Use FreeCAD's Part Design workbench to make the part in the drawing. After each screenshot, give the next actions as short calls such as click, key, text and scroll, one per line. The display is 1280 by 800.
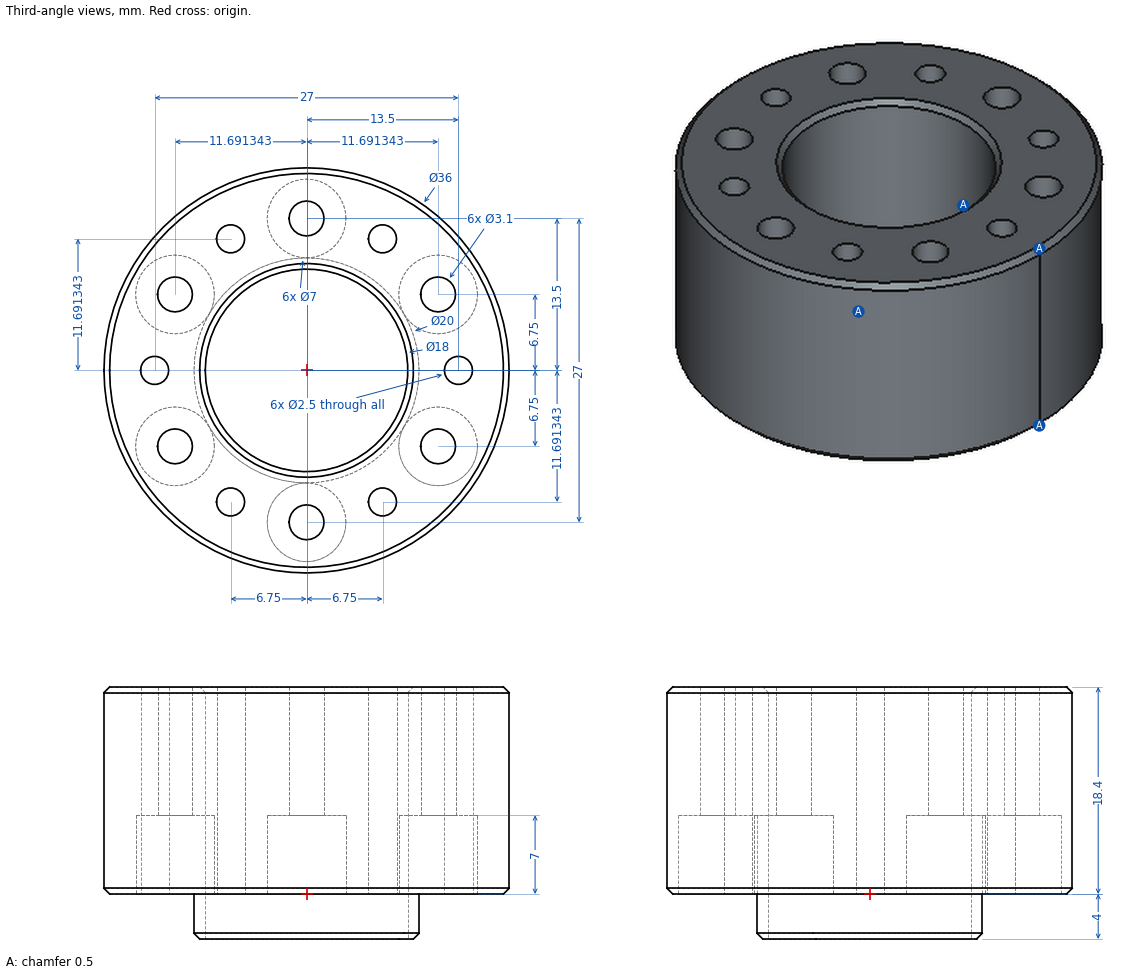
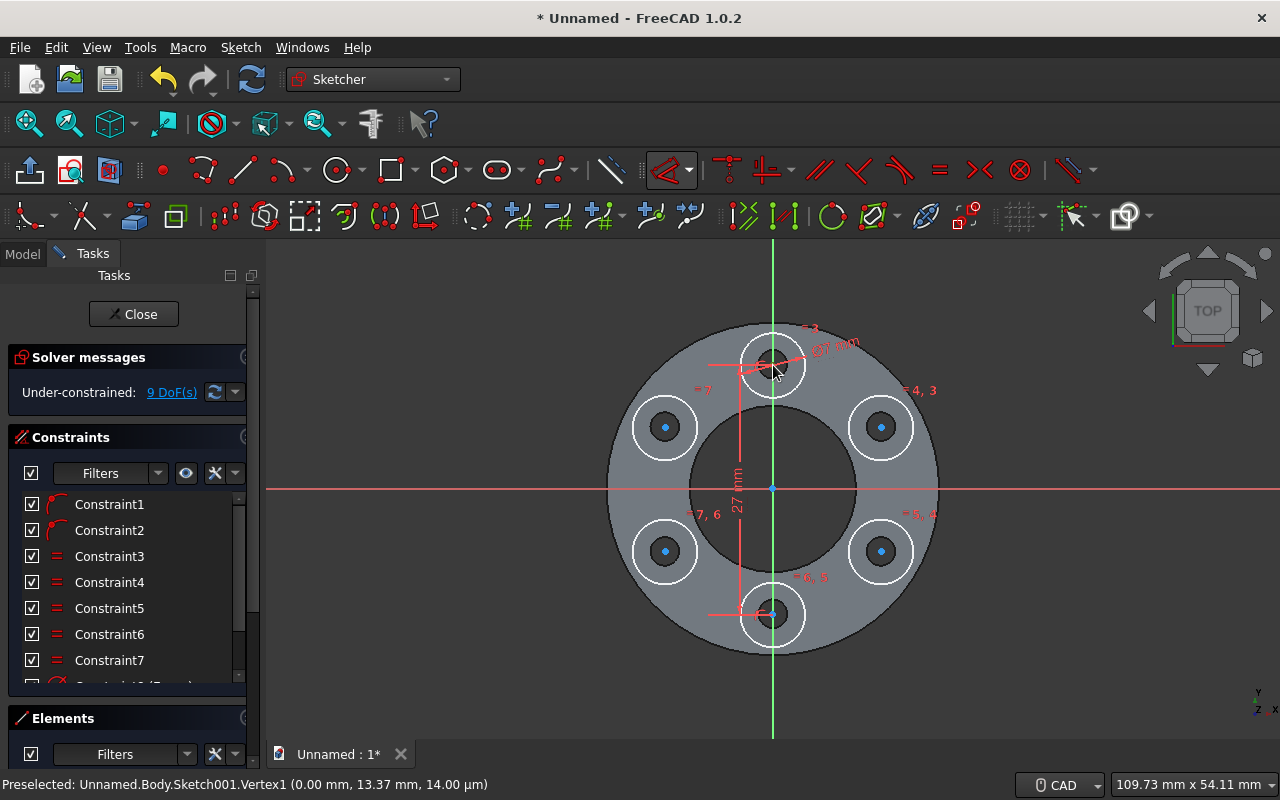
key(i)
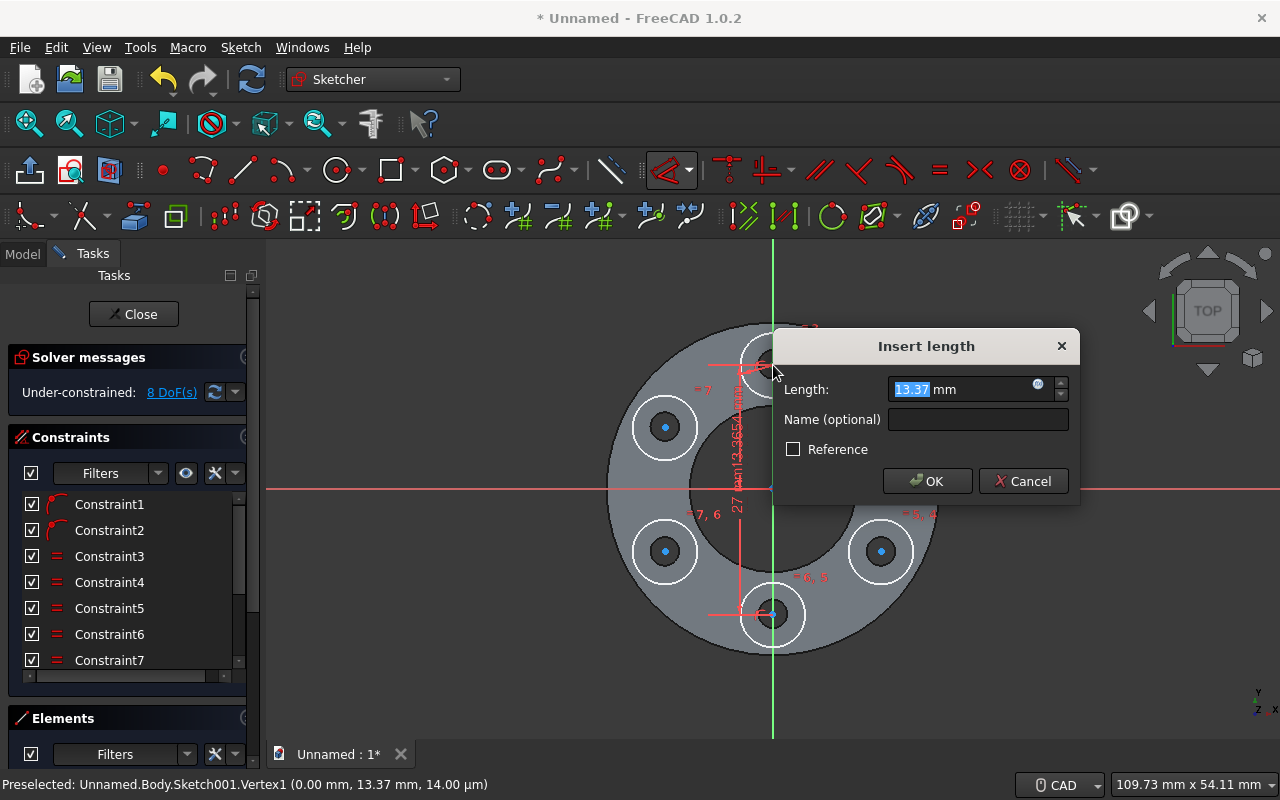
text(13.5)
key(Return)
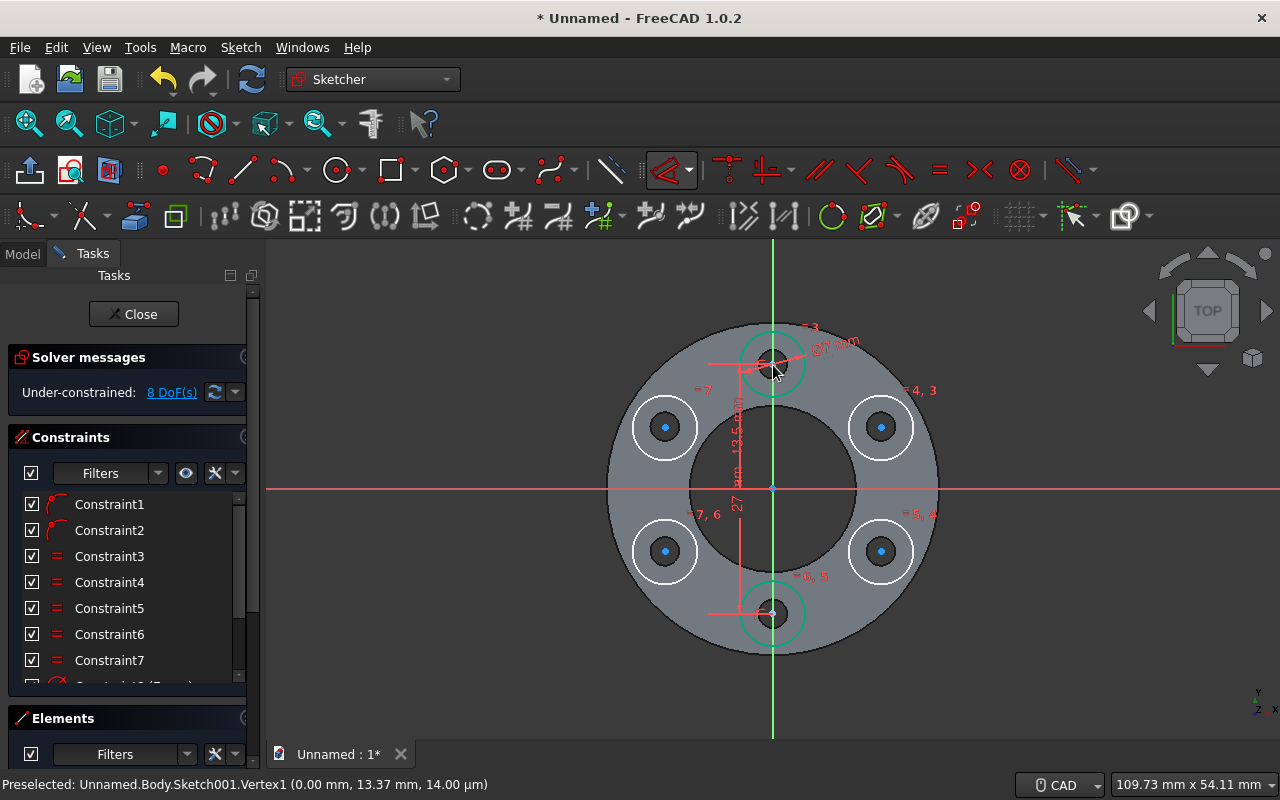
click(881, 428)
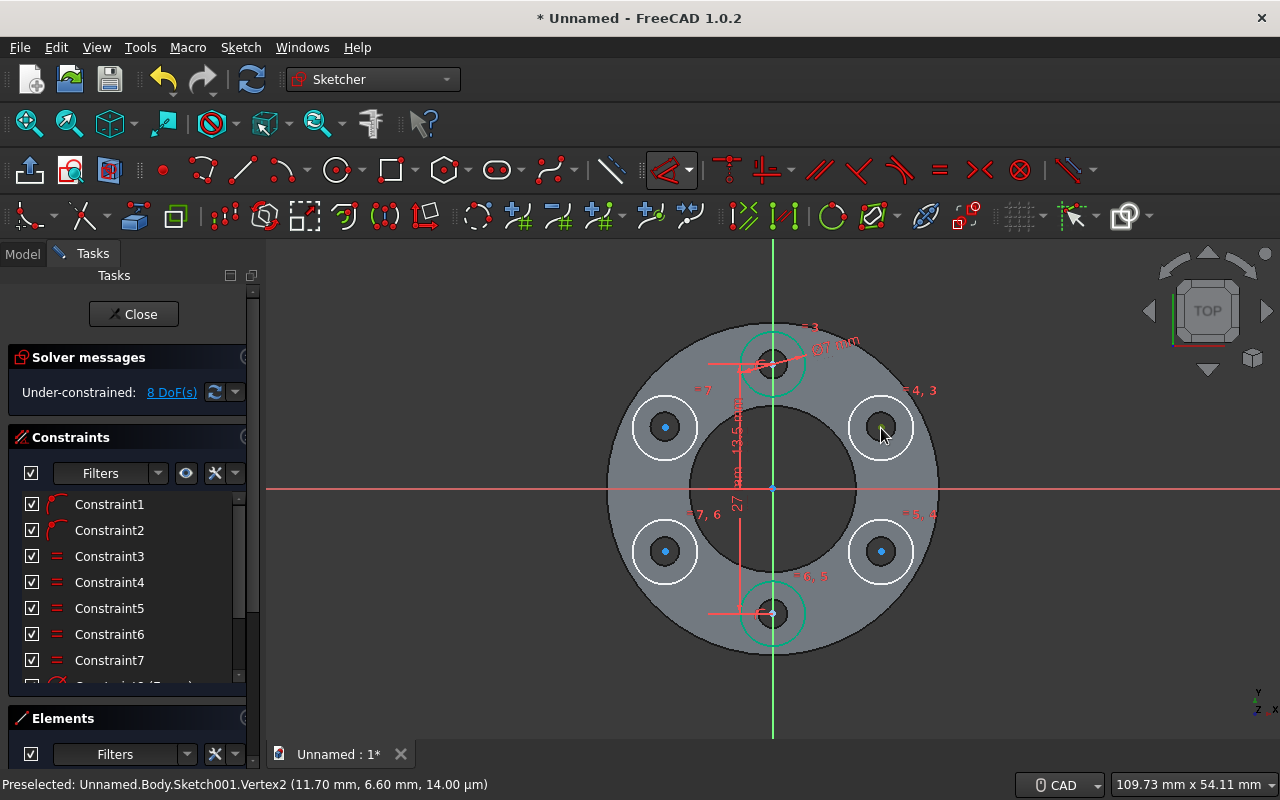
click(692, 170)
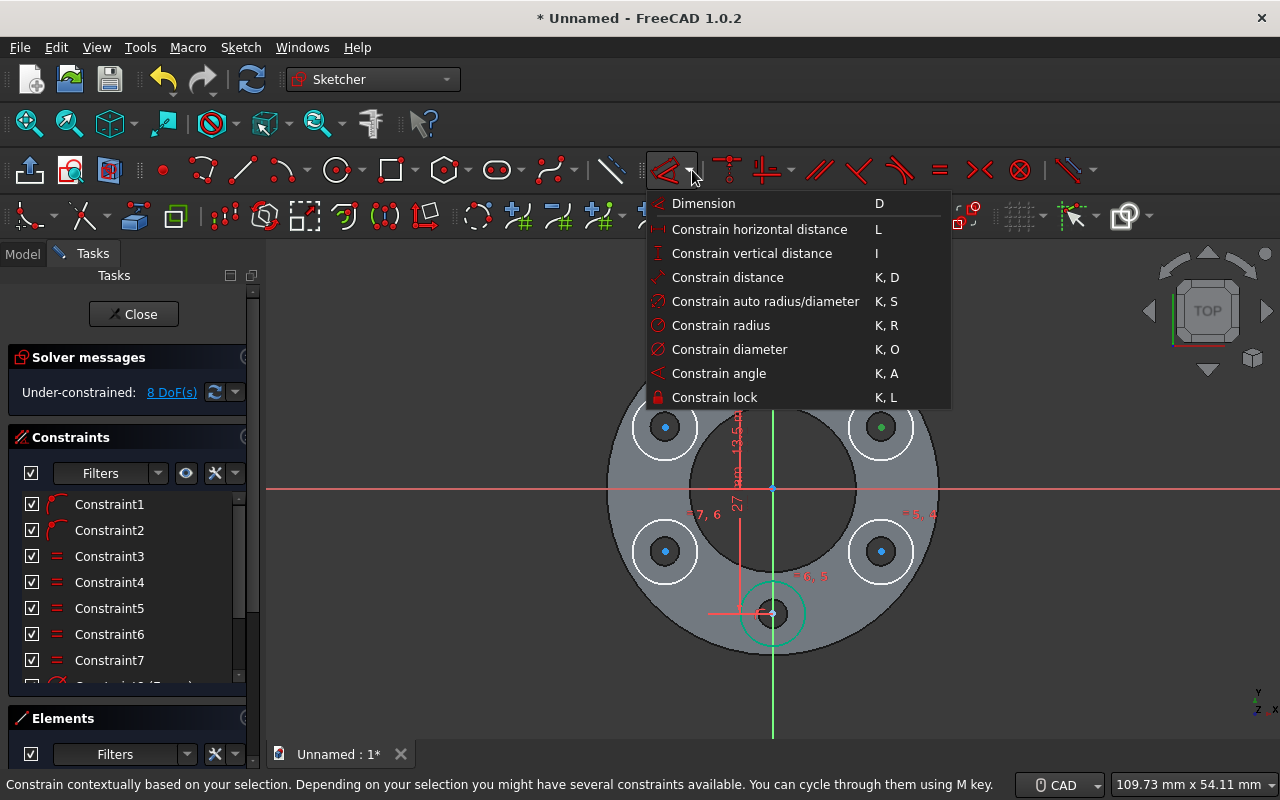
click(799, 253)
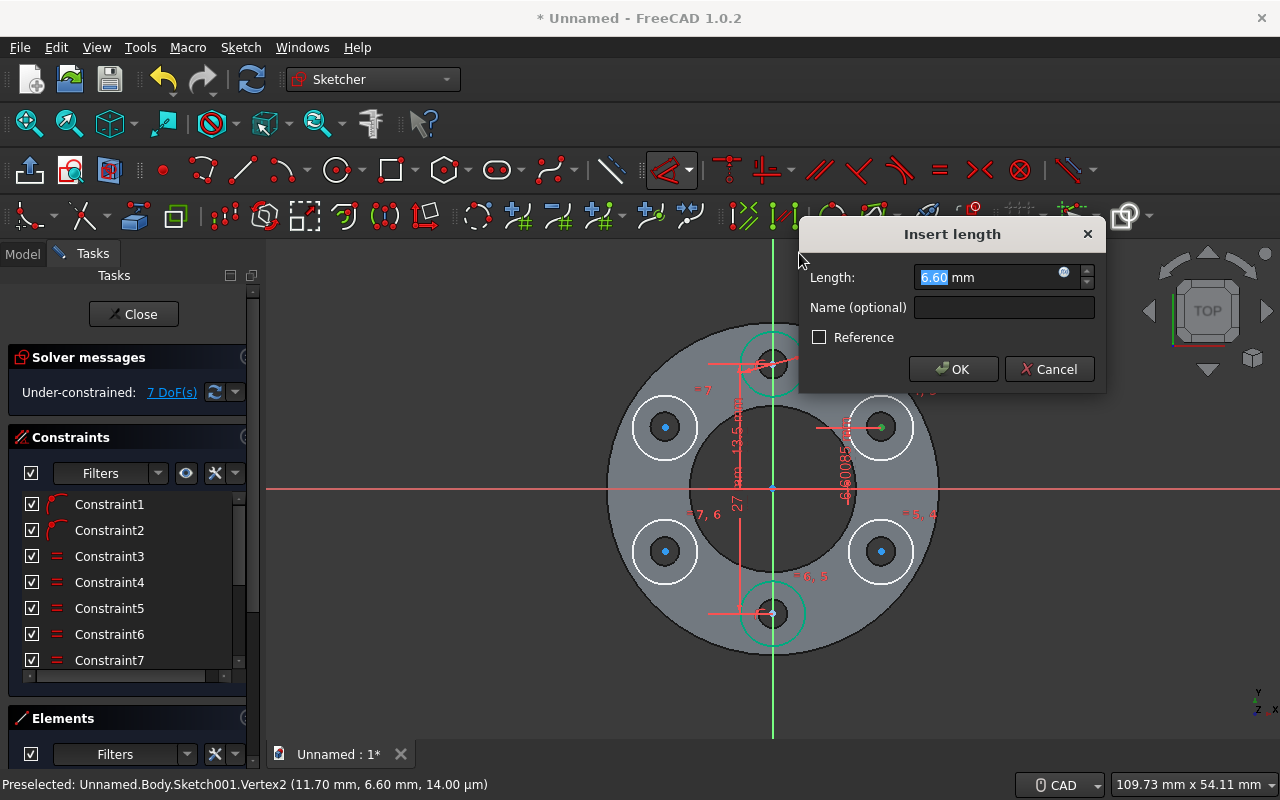
text(6.75)
key(Return)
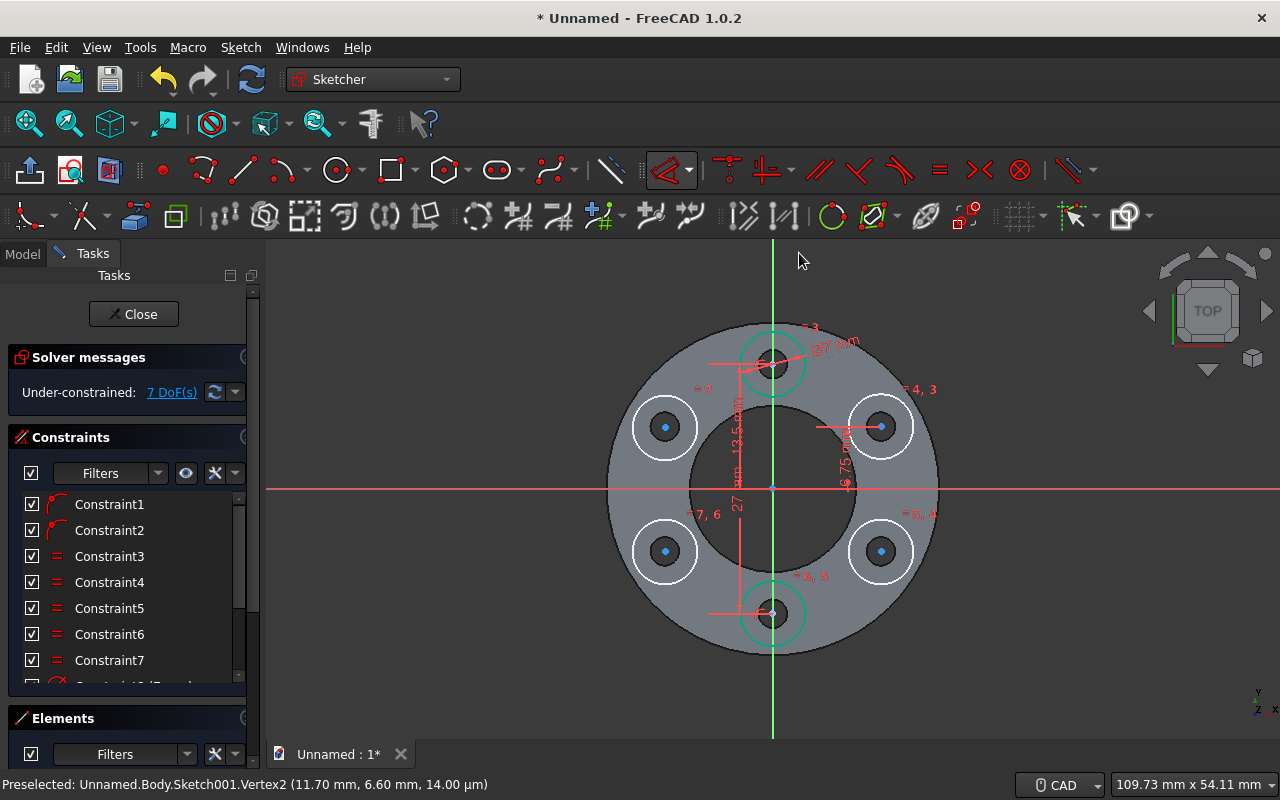
click(881, 552)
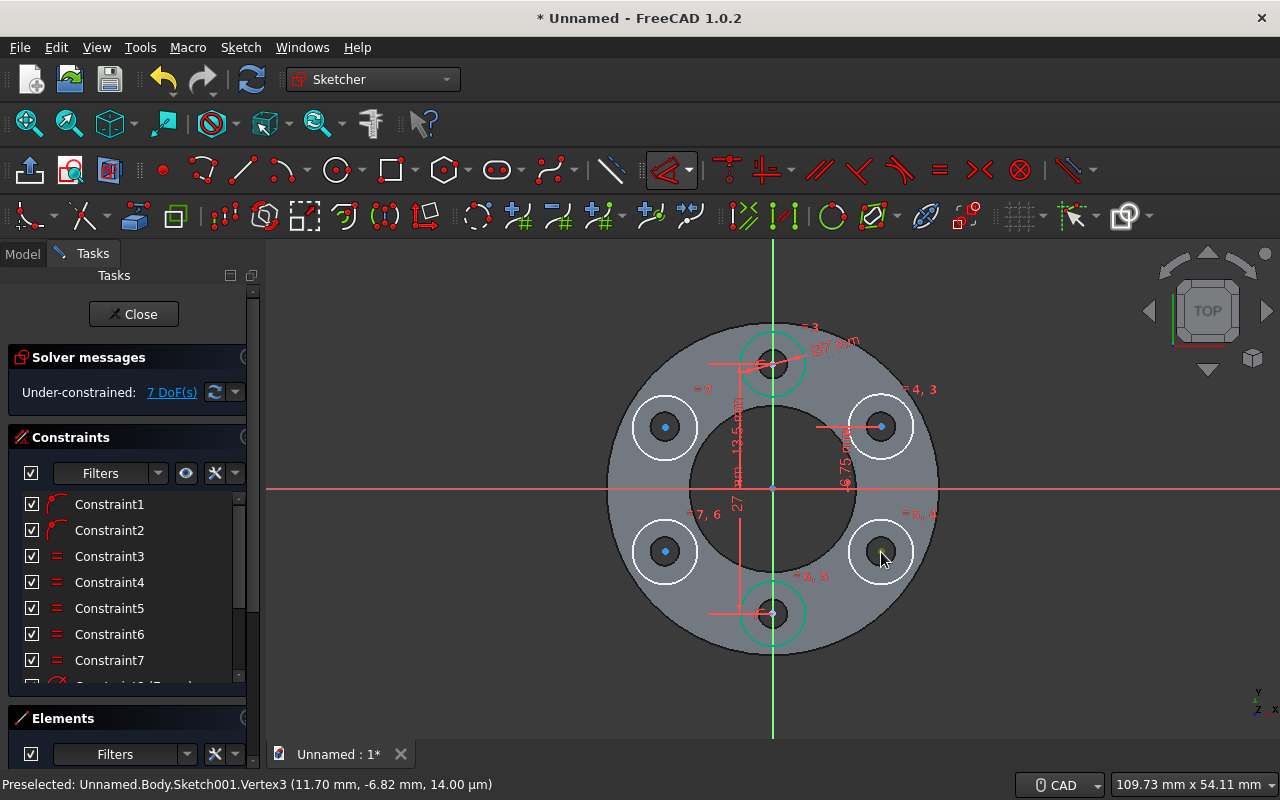
key(i)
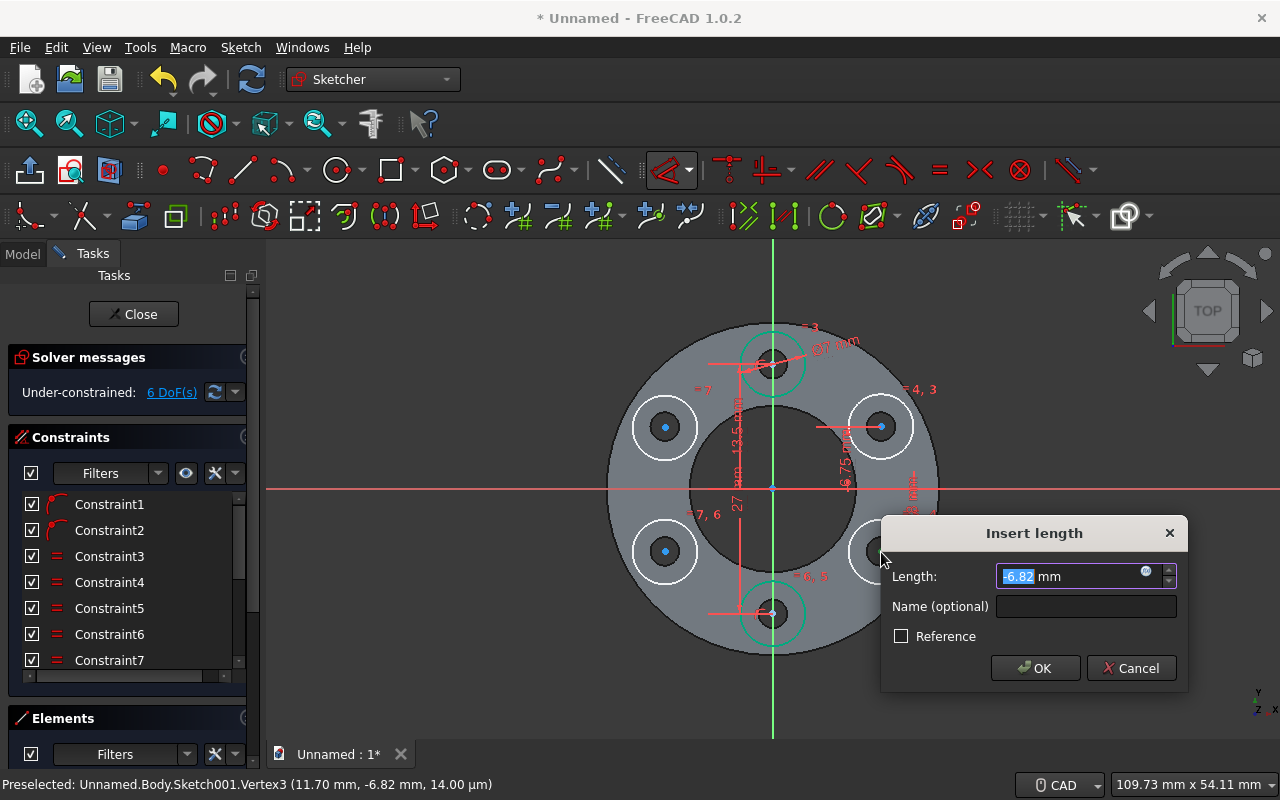
text(-6.75)
key(Return)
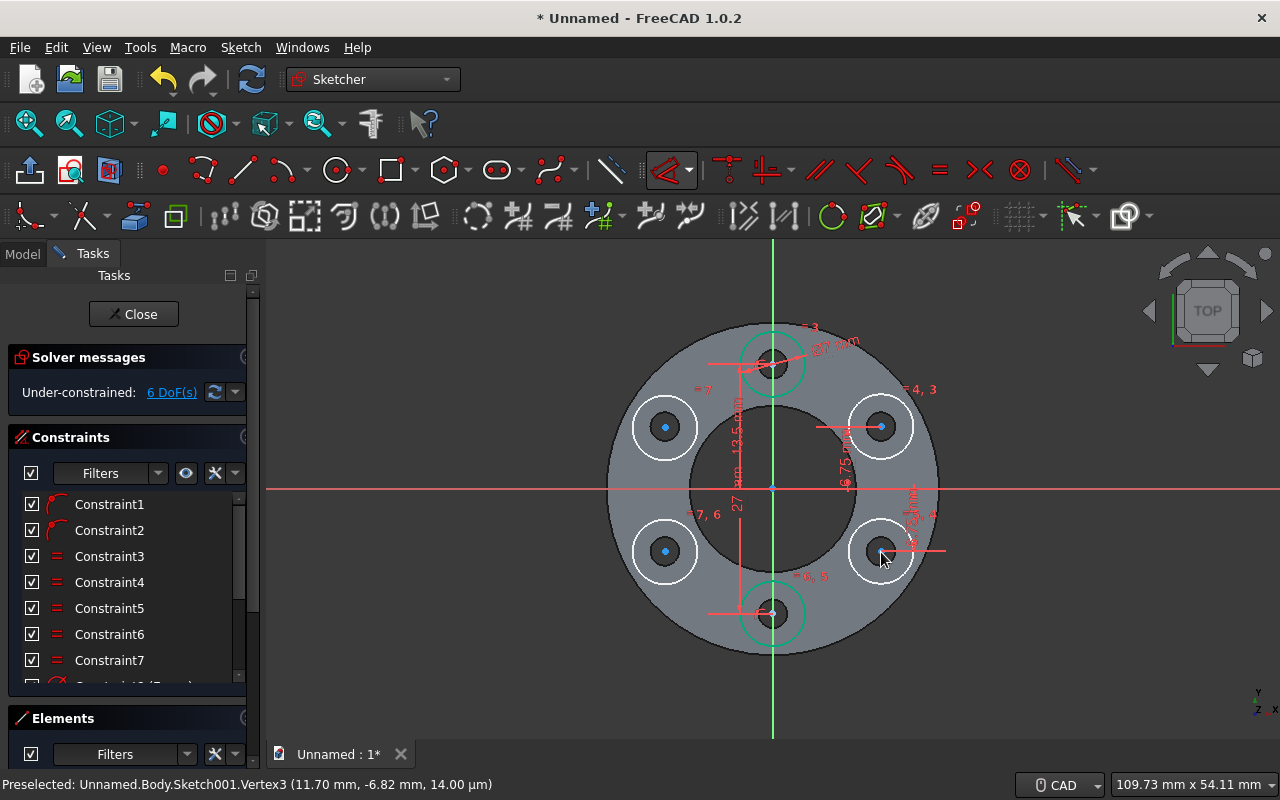
click(665, 552)